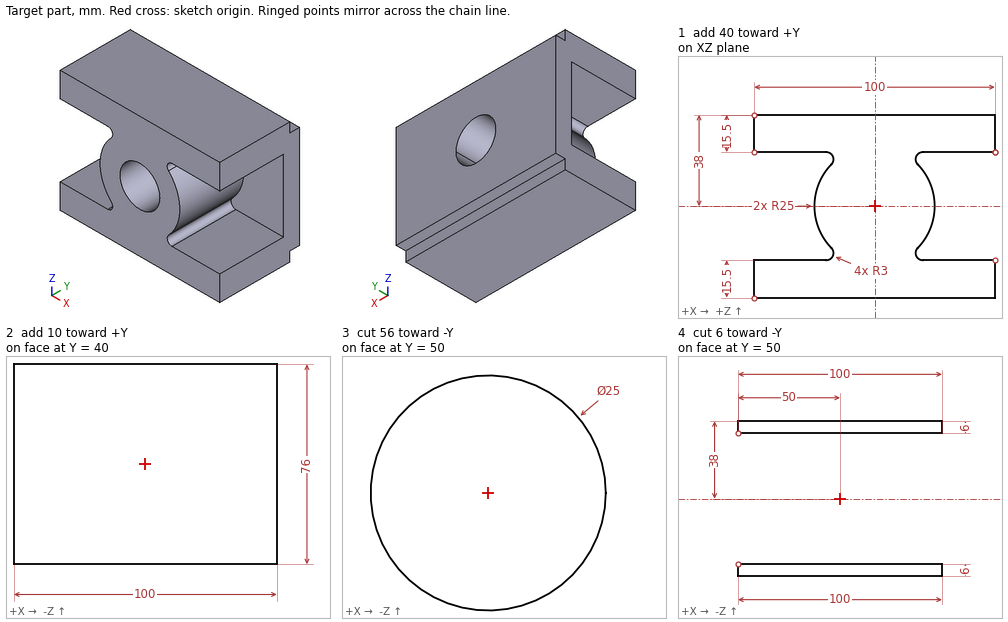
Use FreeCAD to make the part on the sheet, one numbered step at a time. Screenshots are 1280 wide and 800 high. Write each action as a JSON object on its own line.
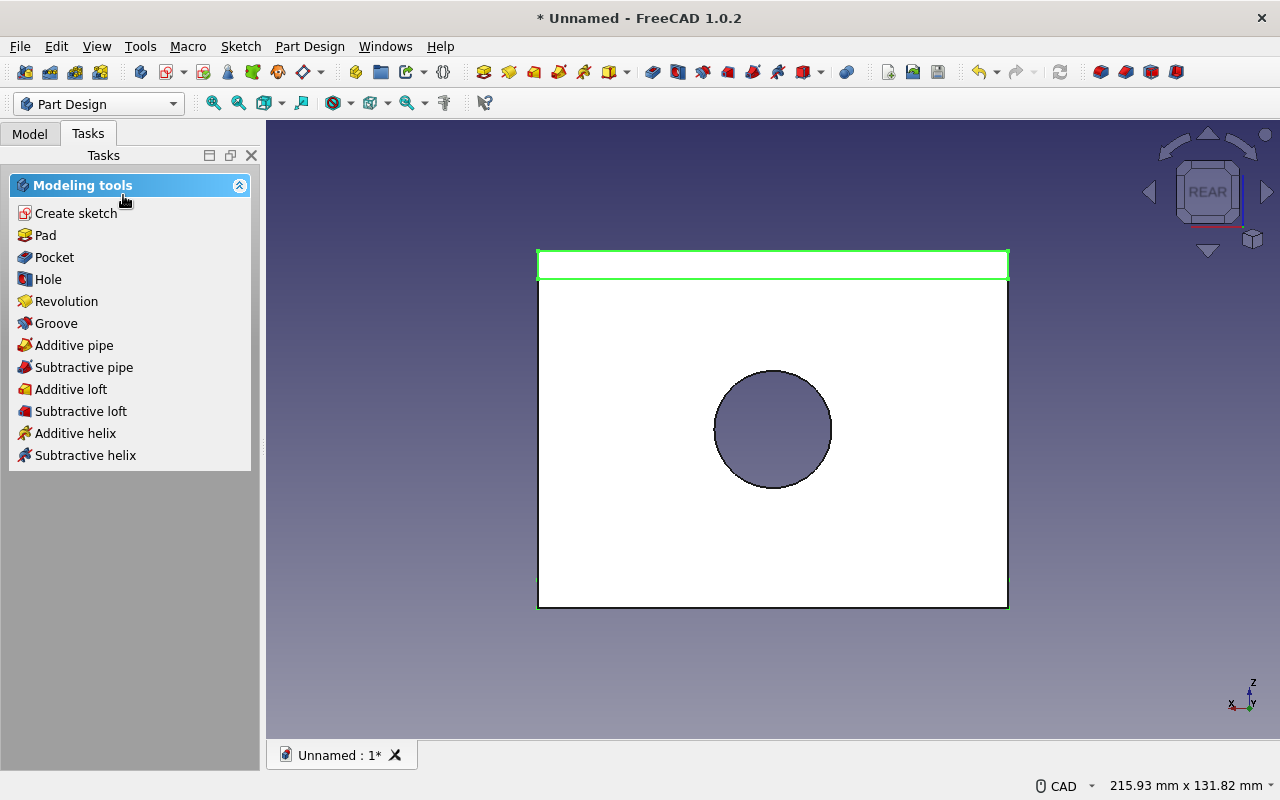
{"action": "left_click", "coordinate": [653, 72]}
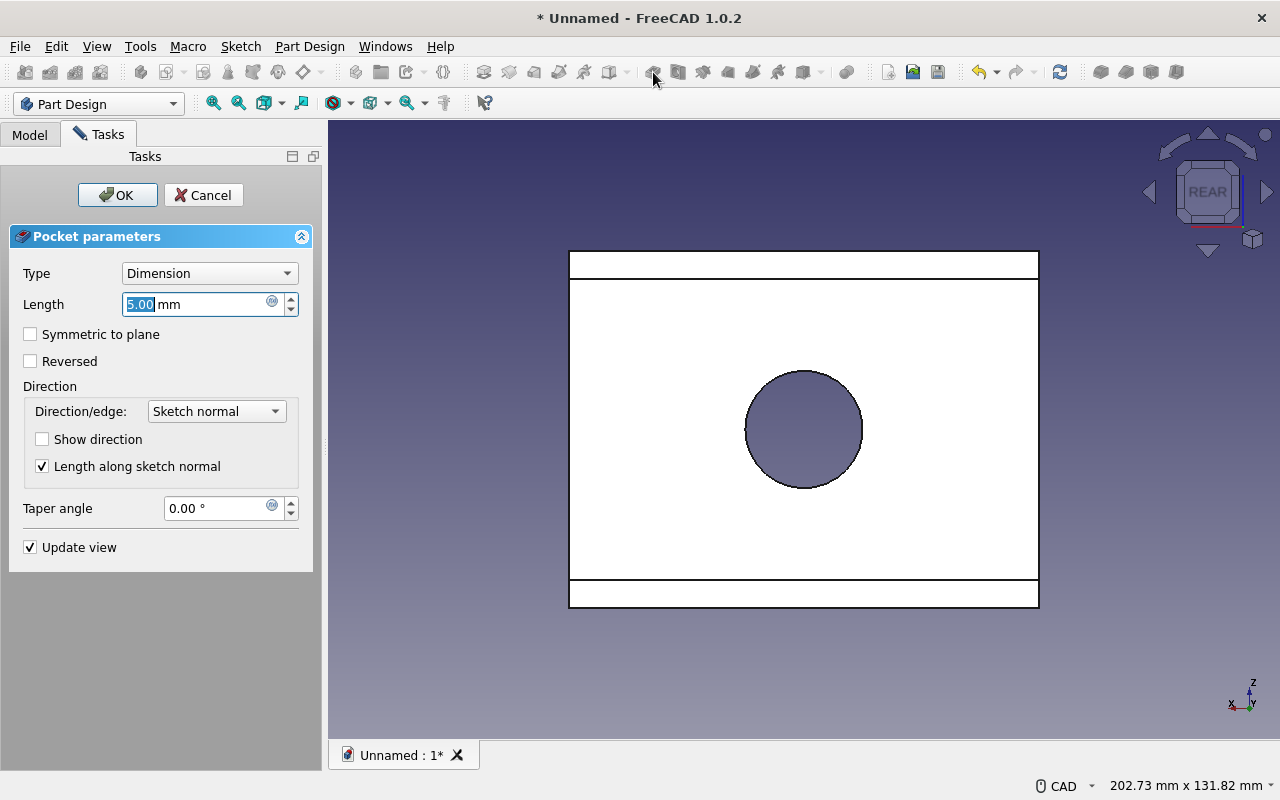
{"action": "type", "text": "6"}
{"action": "key", "text": "Tab"}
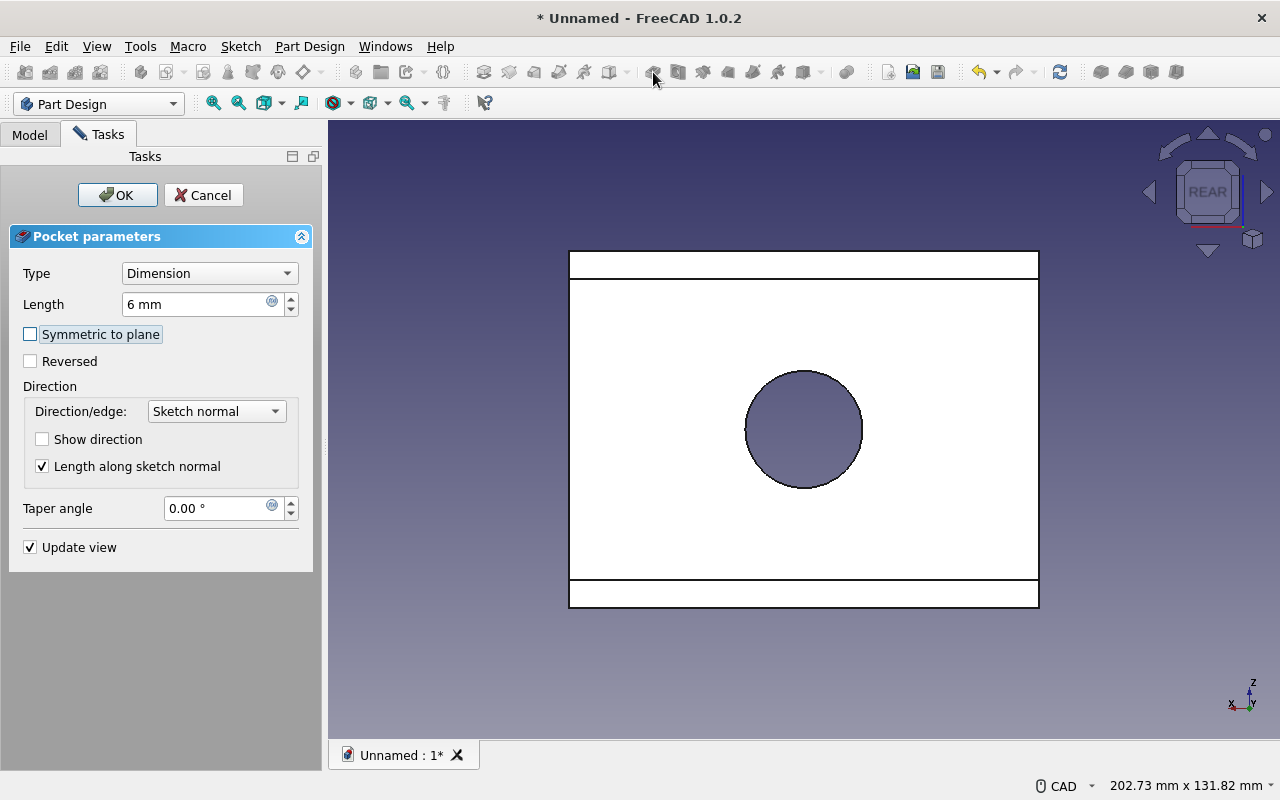
{"action": "left_click", "coordinate": [118, 195]}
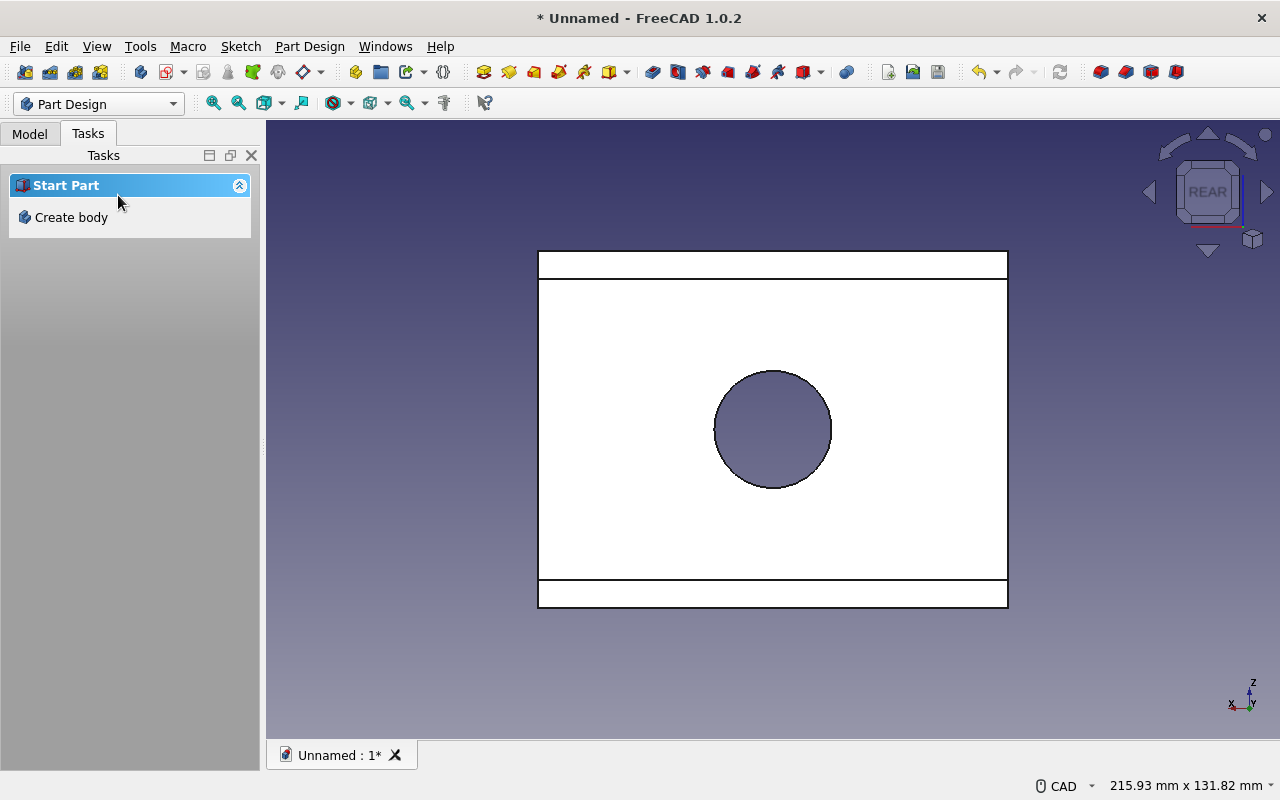
{"action": "key", "text": "0"}